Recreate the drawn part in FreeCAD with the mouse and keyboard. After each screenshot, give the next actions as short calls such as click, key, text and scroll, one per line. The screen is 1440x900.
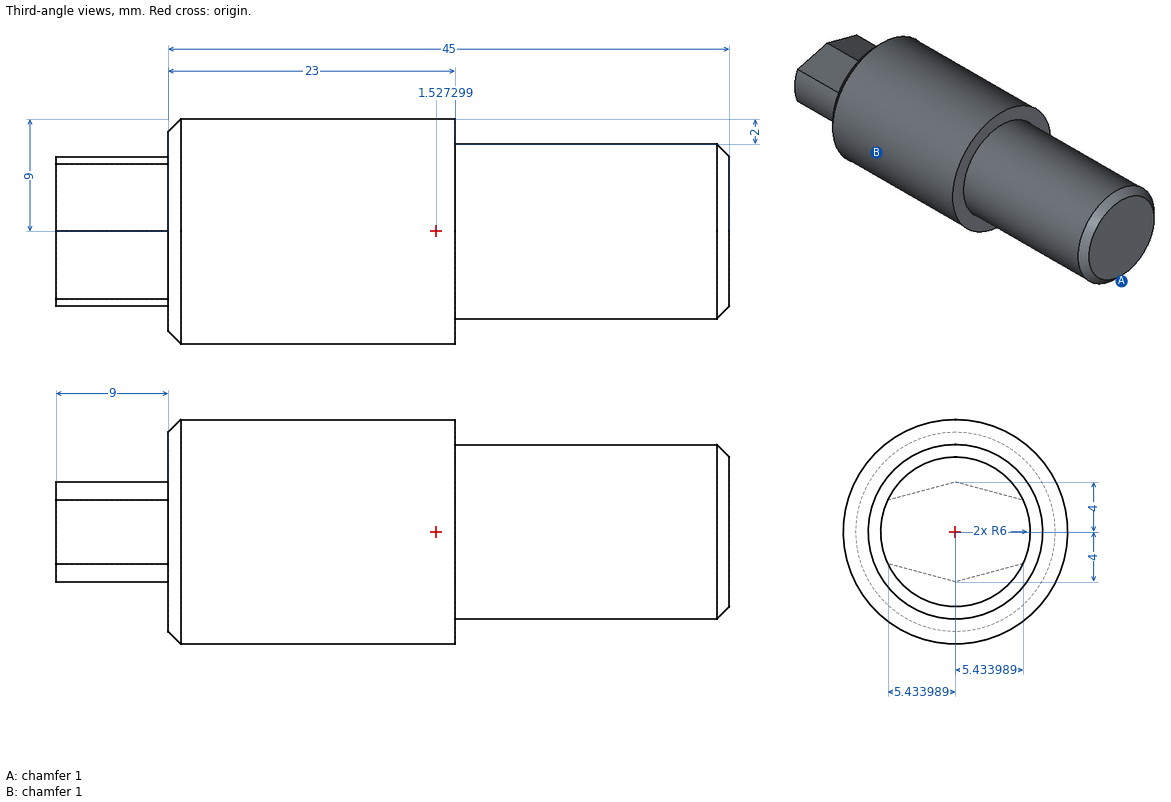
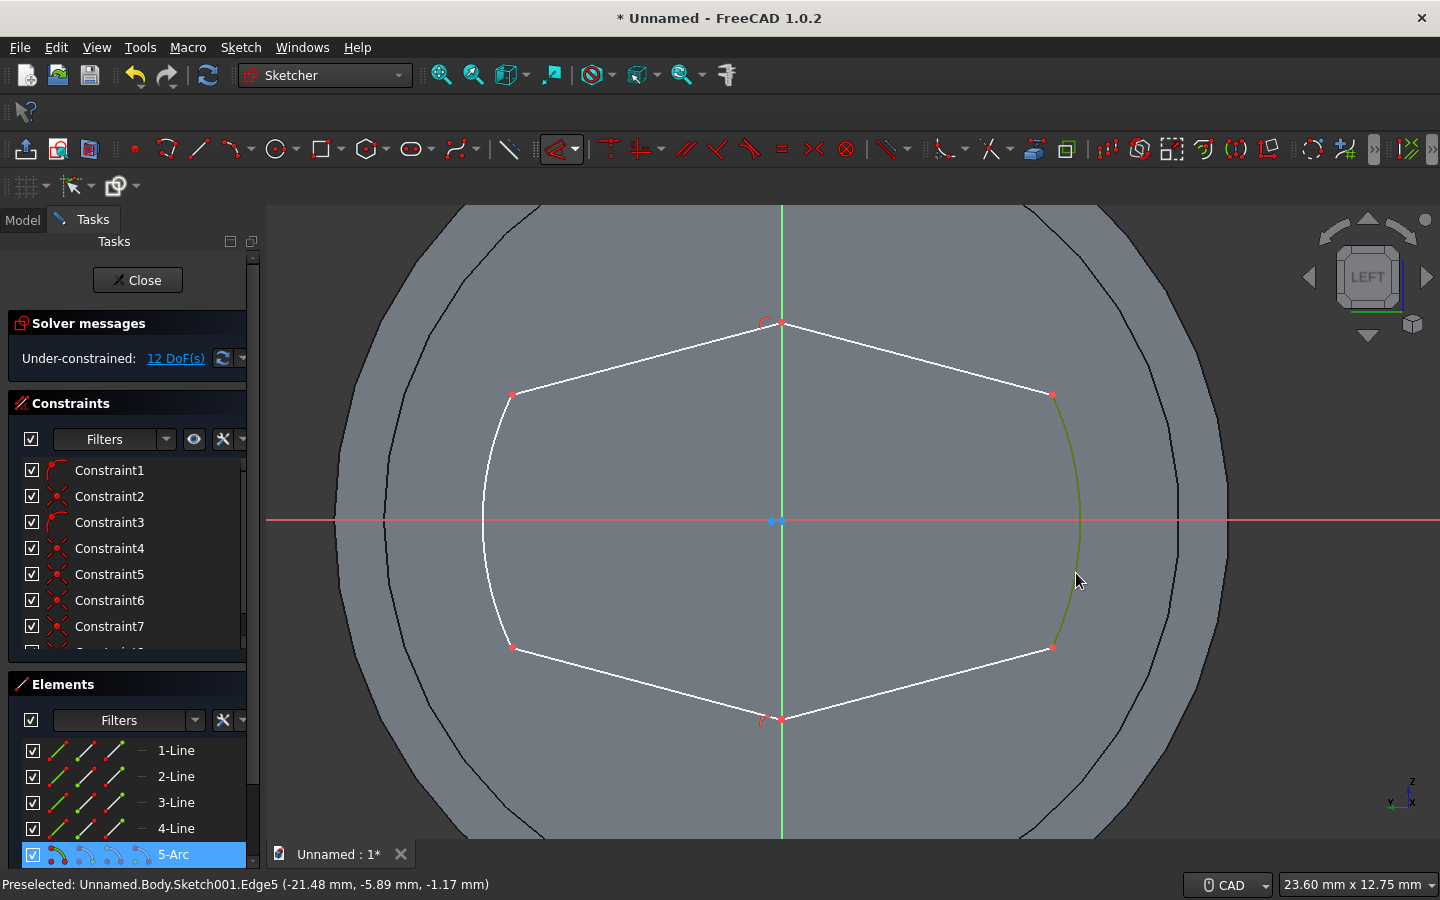
click(488, 469)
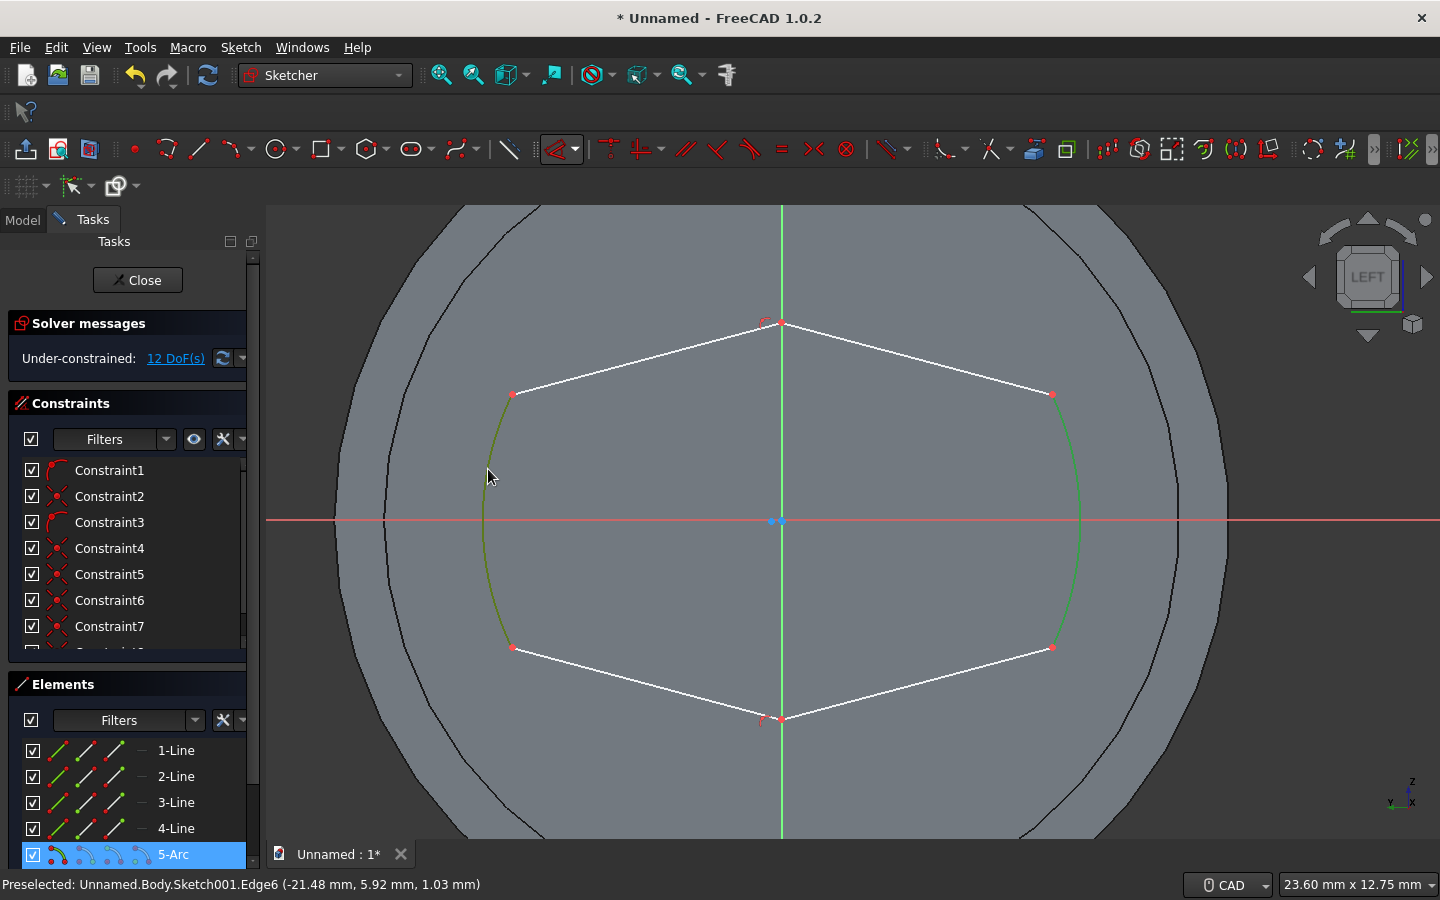
click(610, 150)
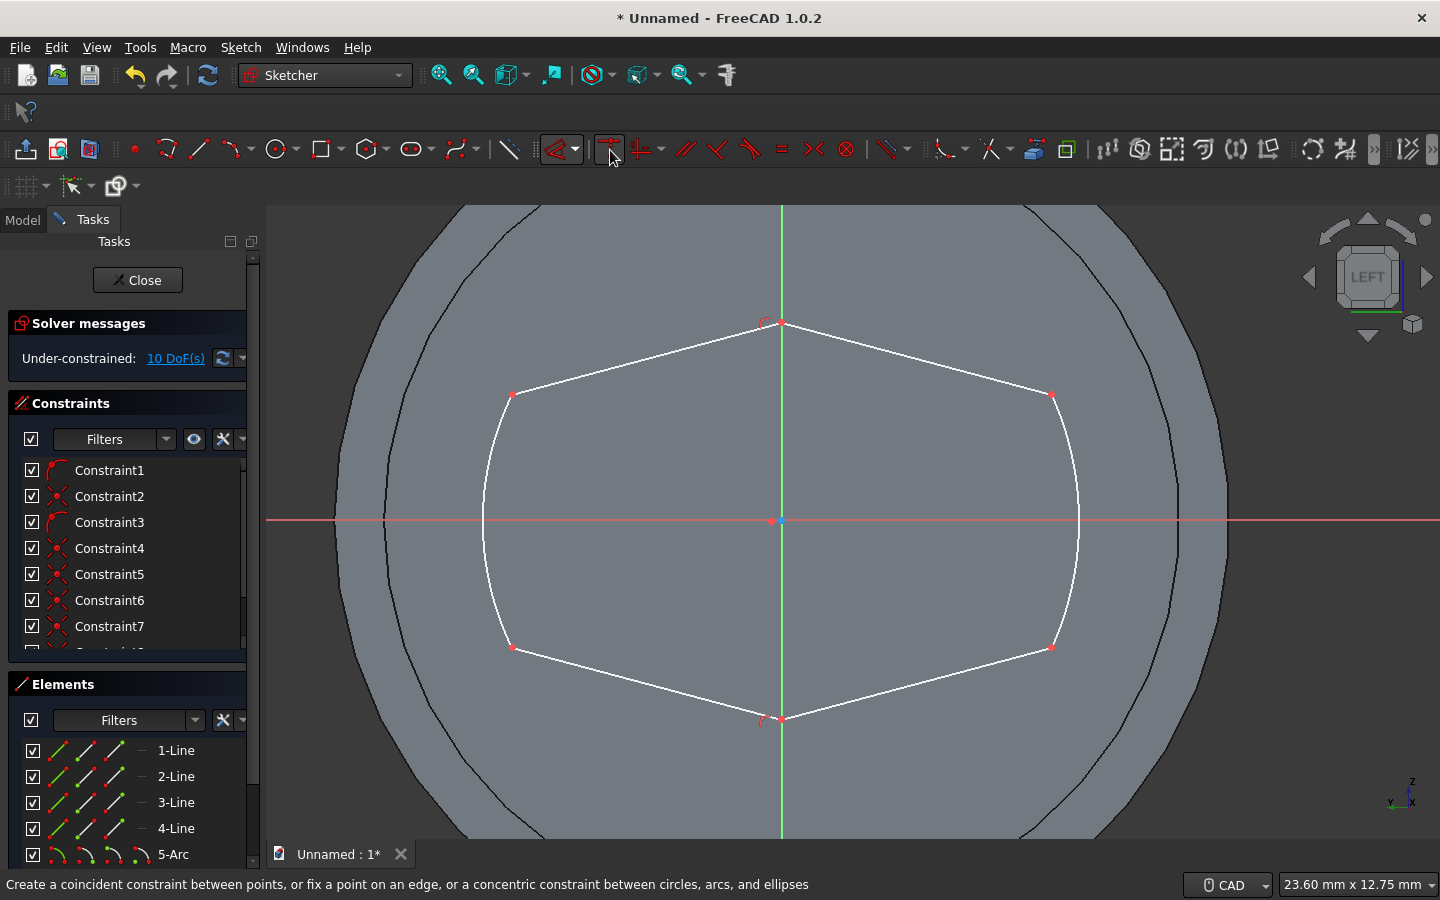
drag(762, 510, 792, 531)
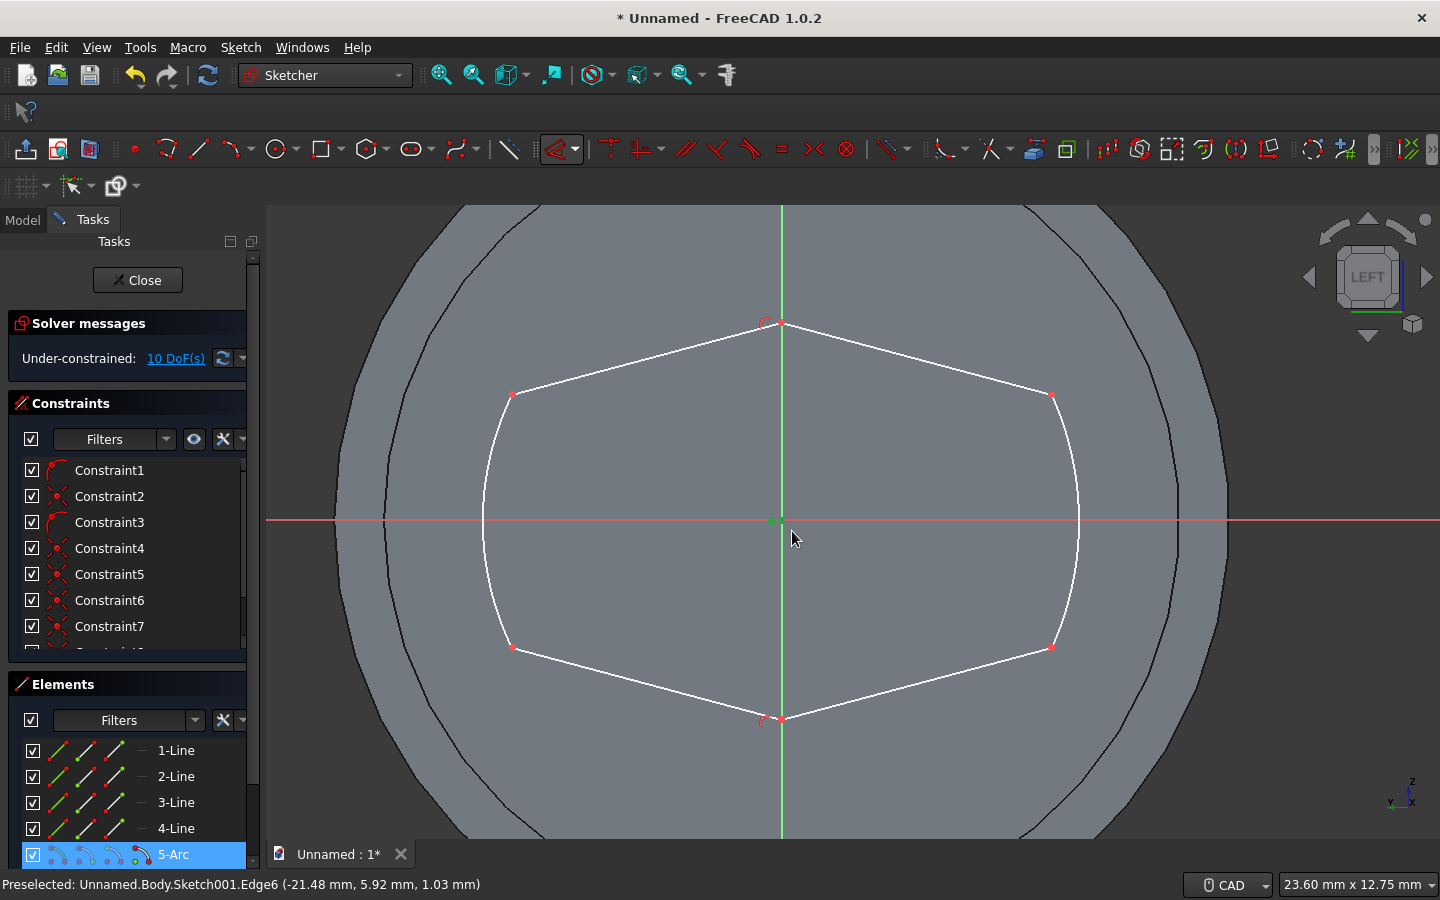
click(610, 150)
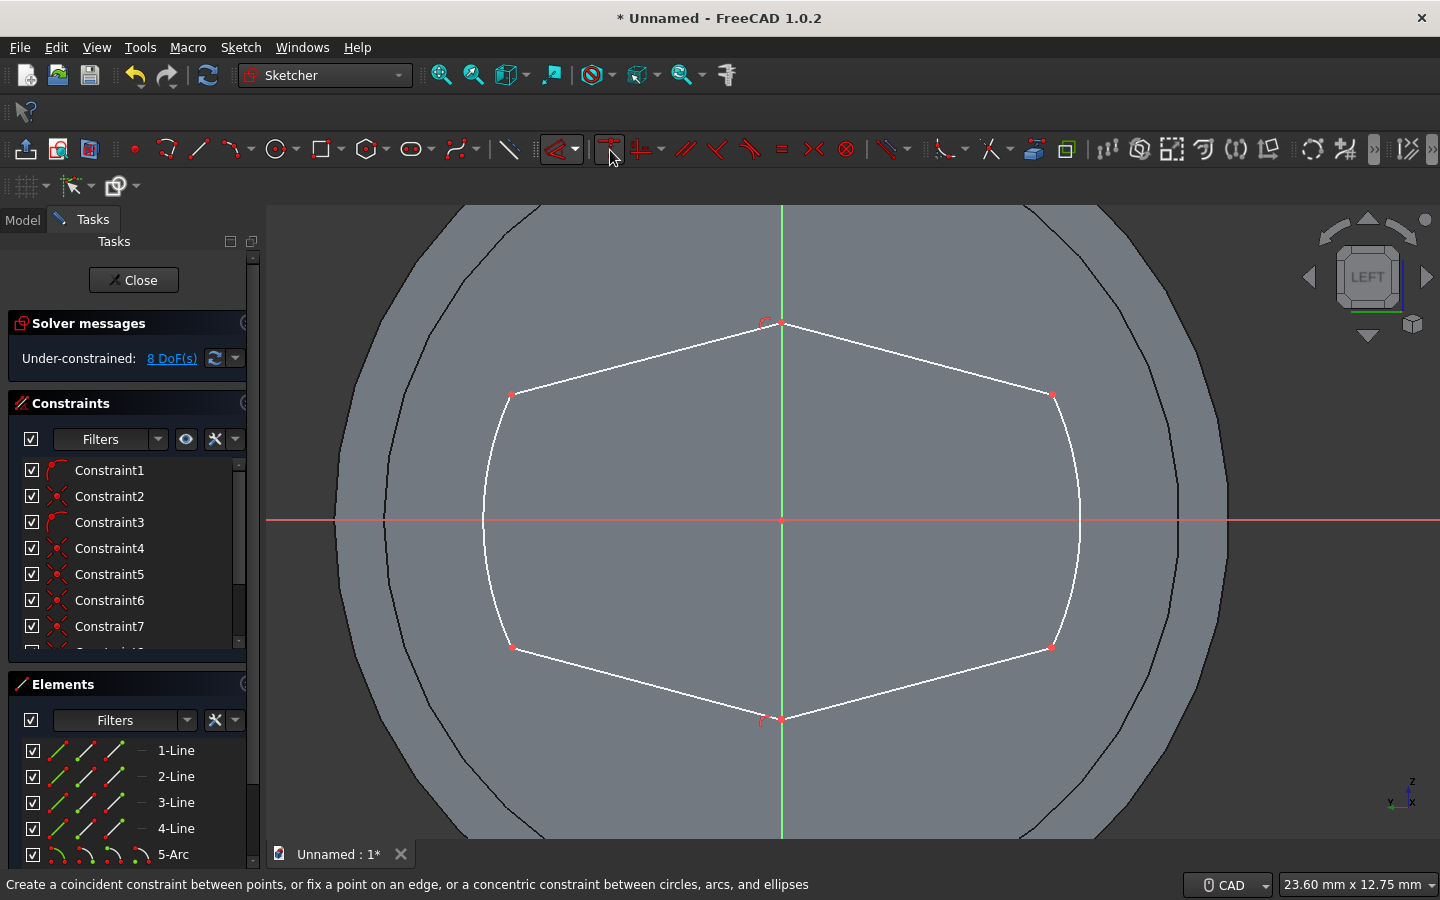
click(1076, 574)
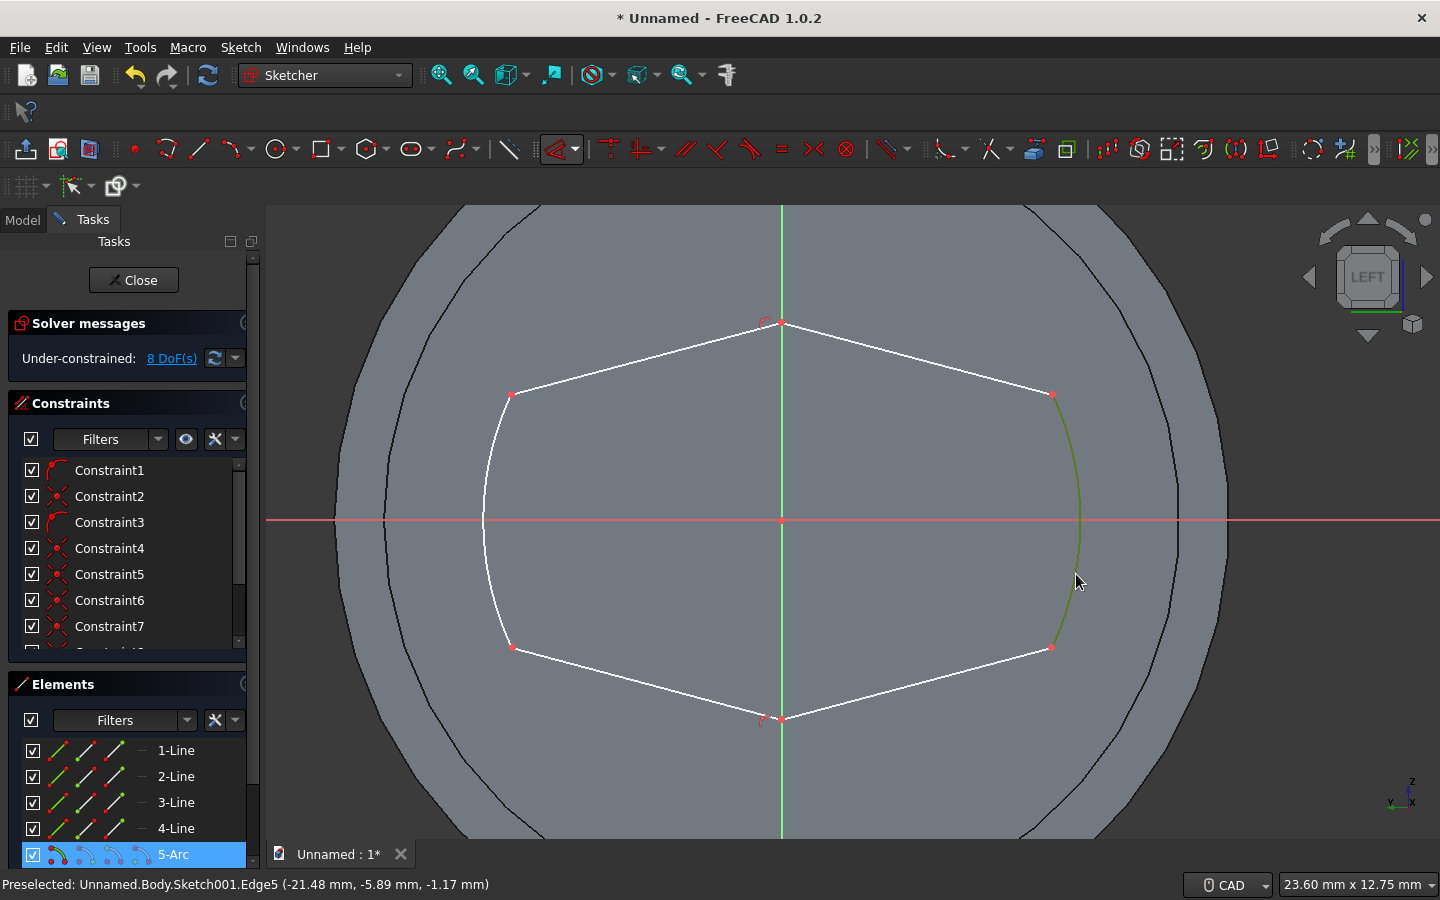
click(488, 470)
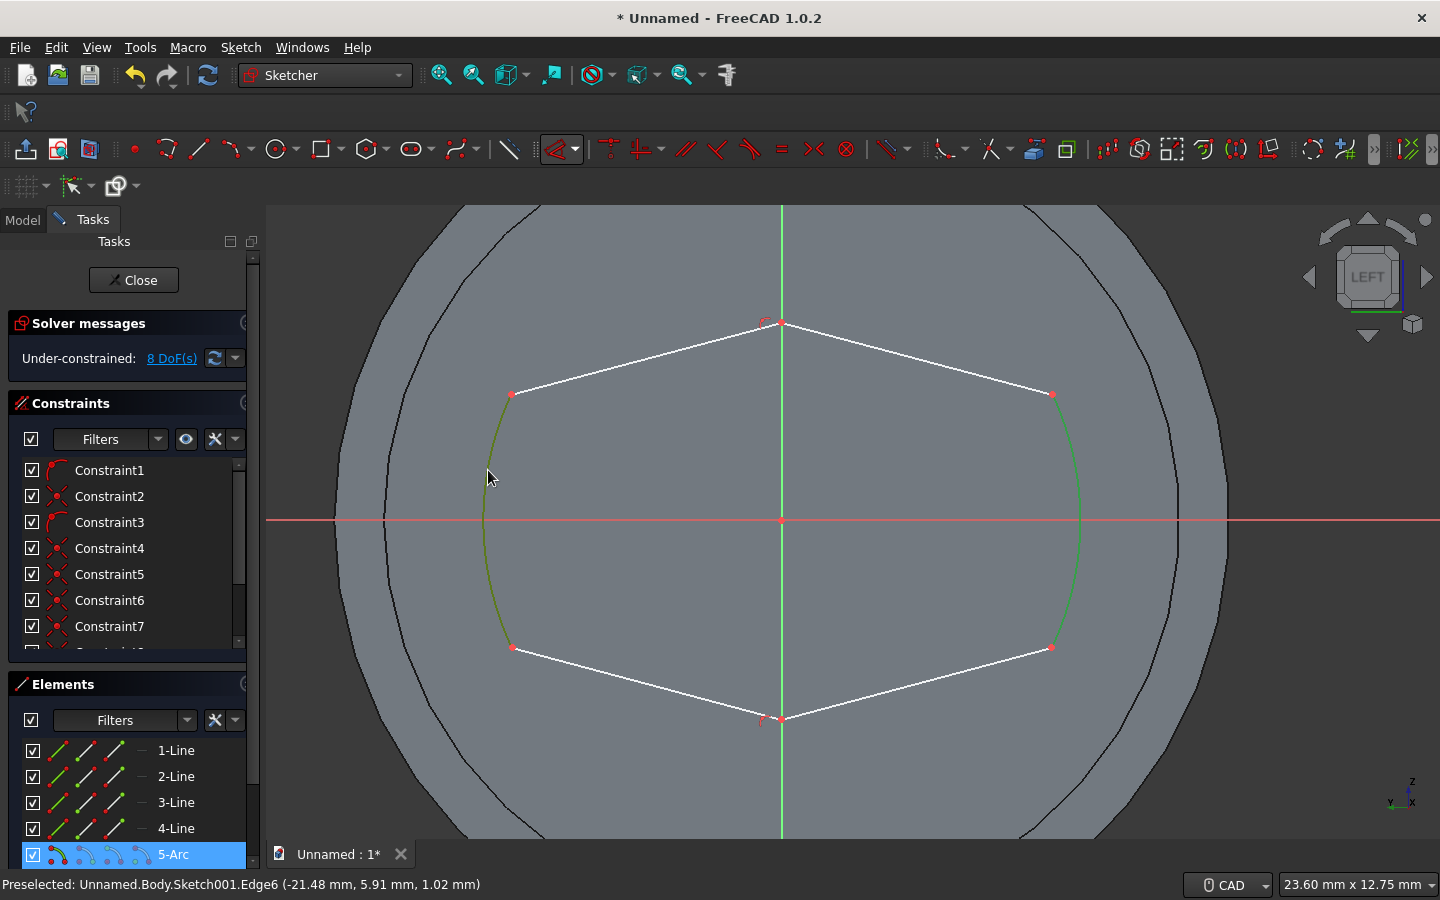
click(782, 150)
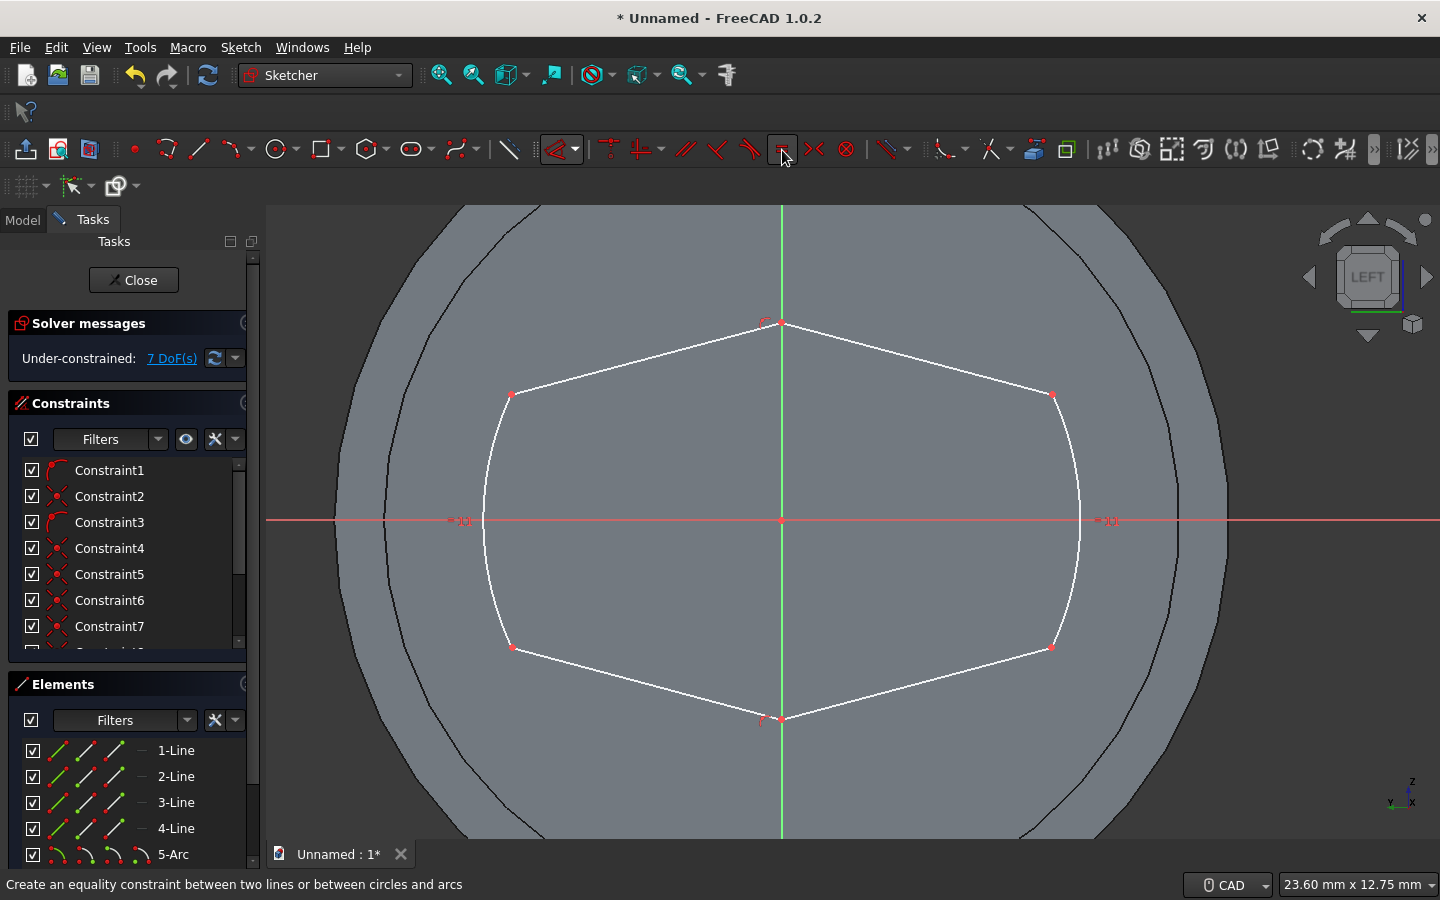
click(1075, 574)